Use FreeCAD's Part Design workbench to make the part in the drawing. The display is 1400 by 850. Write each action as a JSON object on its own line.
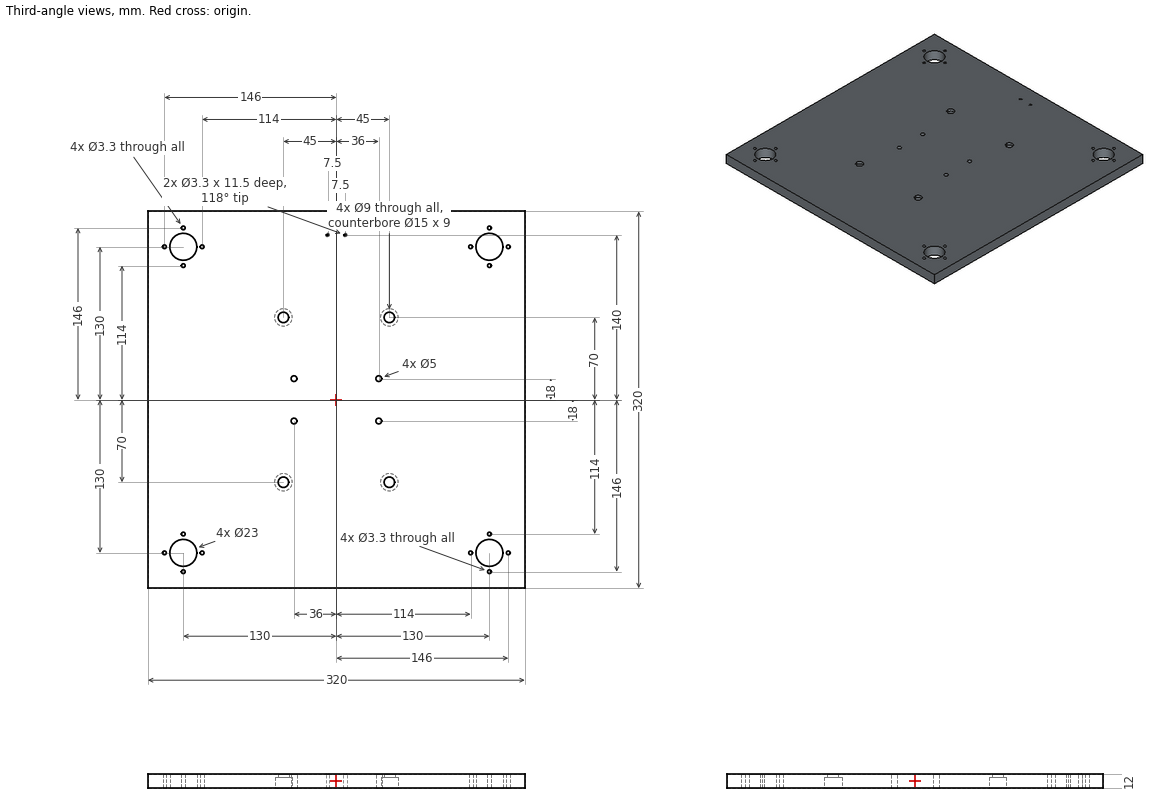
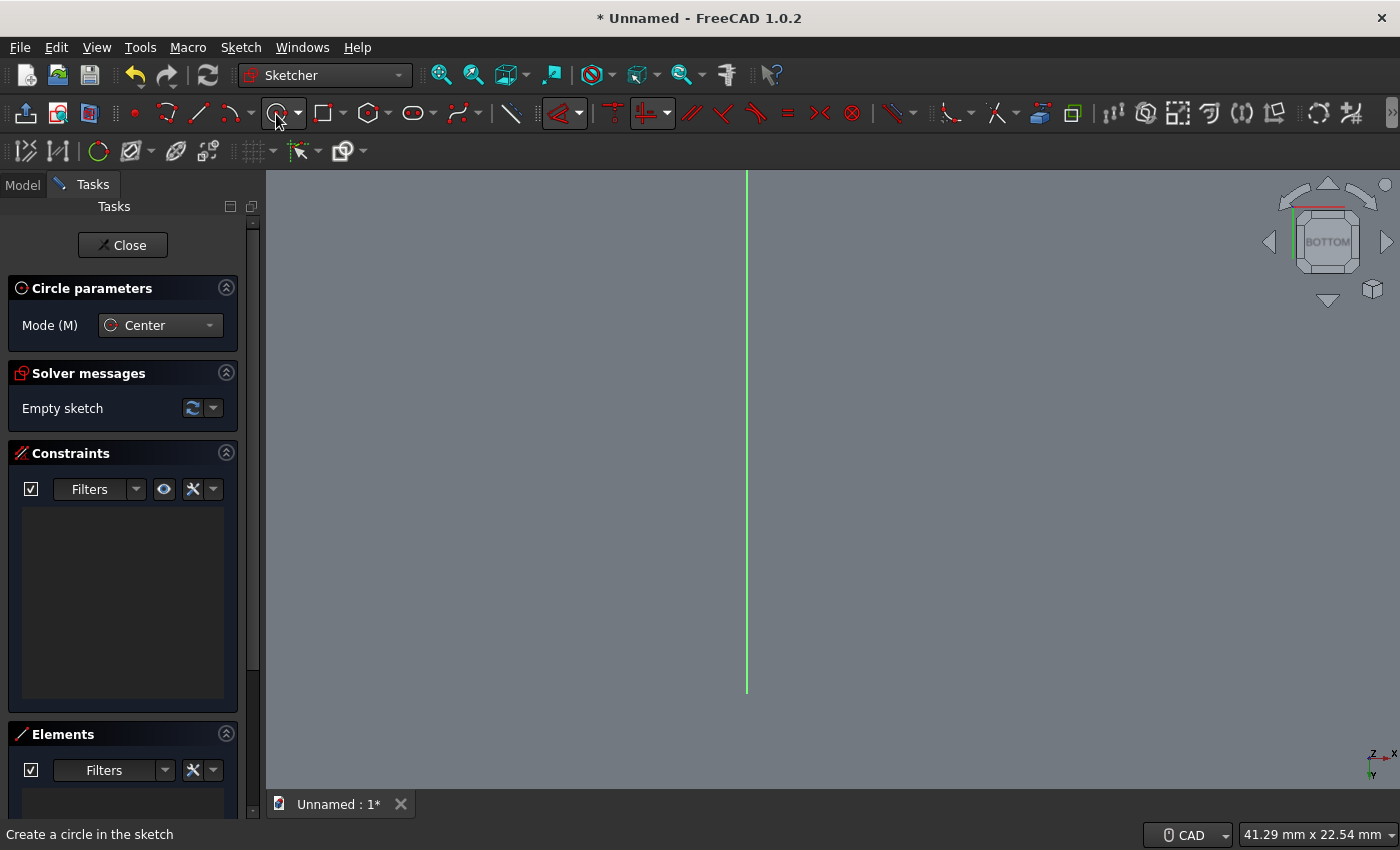
{"action": "left_click", "coordinate": [953, 463]}
{"action": "mouse_move", "coordinate": [985, 431]}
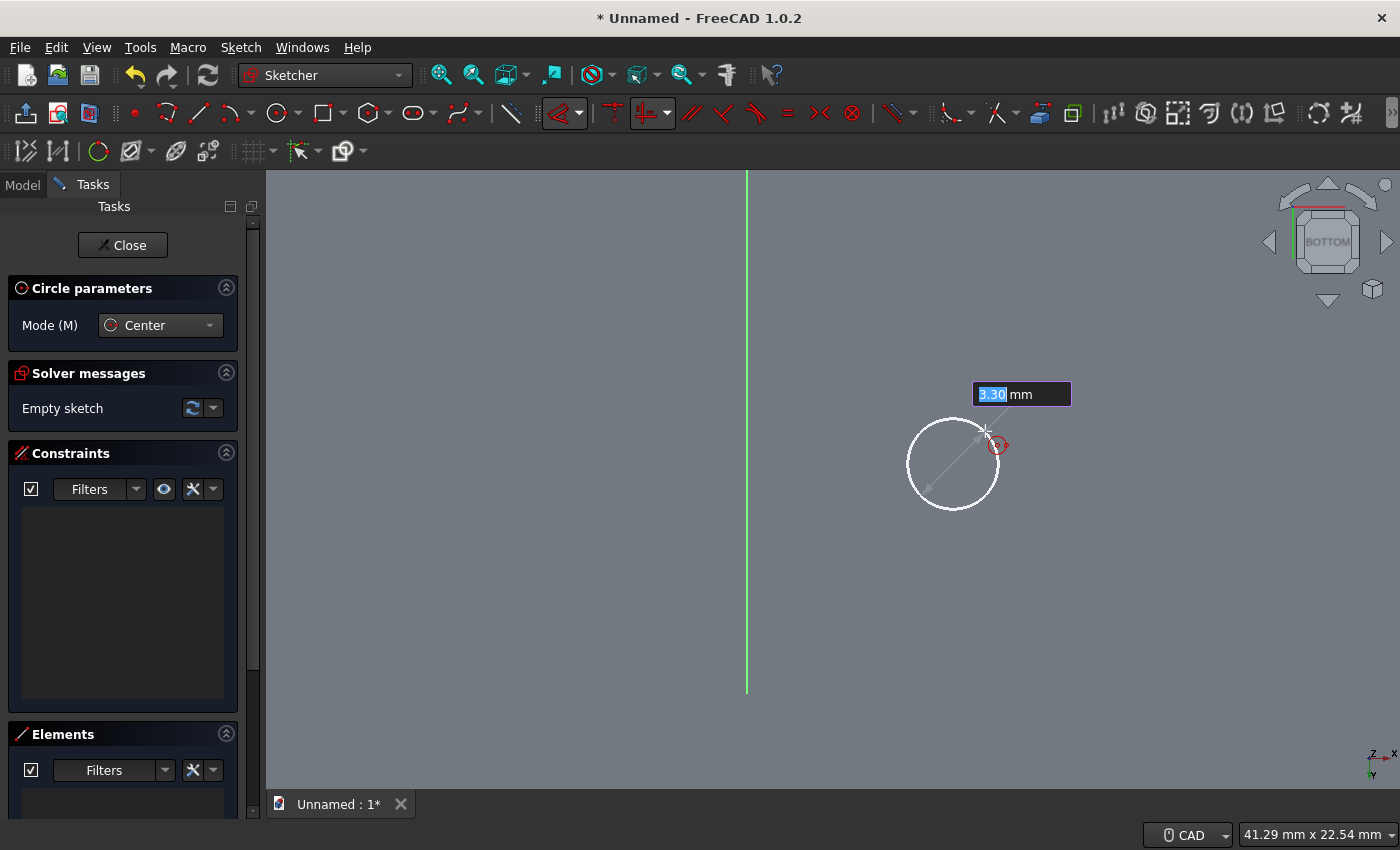
{"action": "type", "text": "3.3"}
{"action": "key", "text": "Return"}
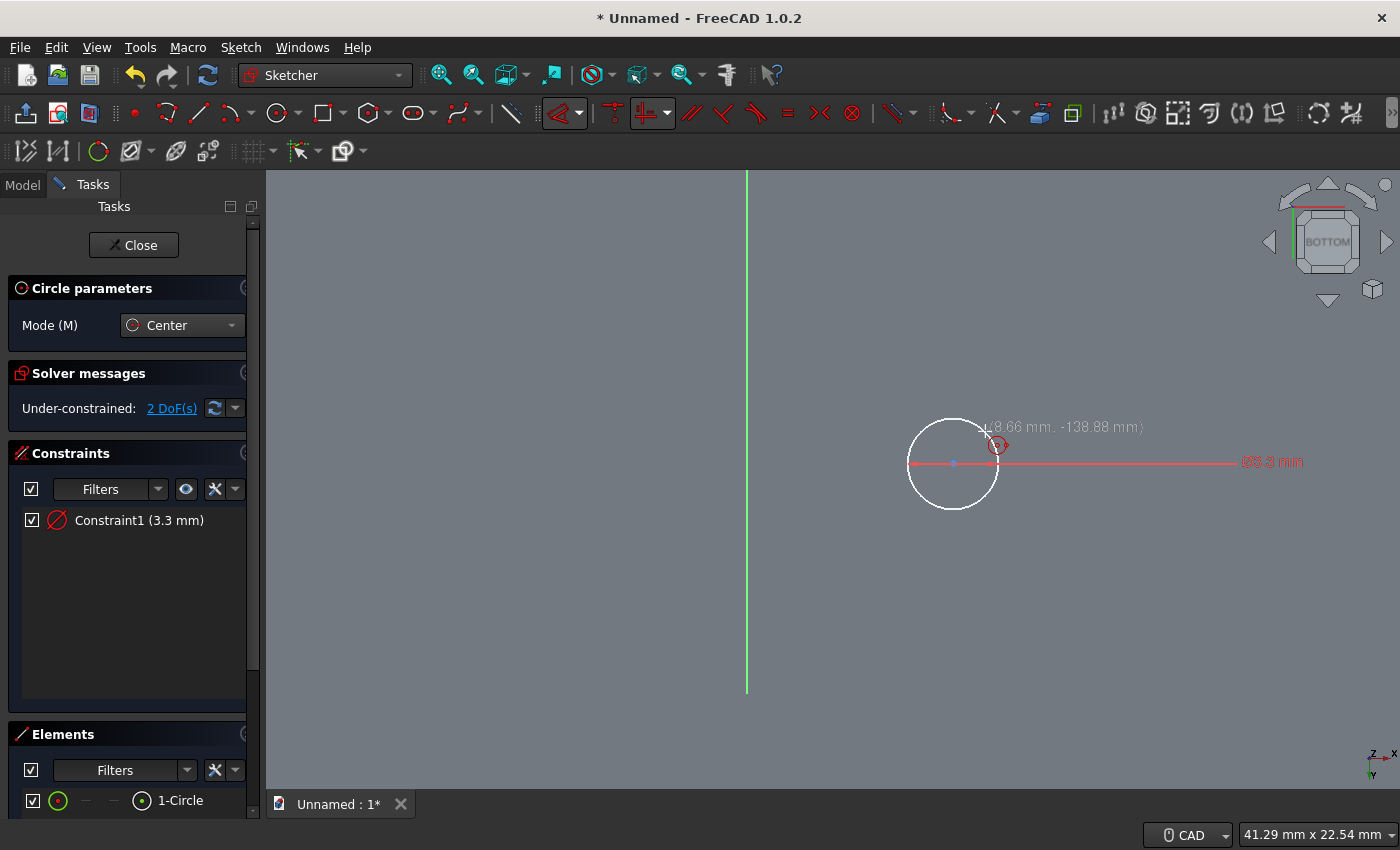
{"action": "left_click", "coordinate": [541, 463]}
{"action": "mouse_move", "coordinate": [573, 431]}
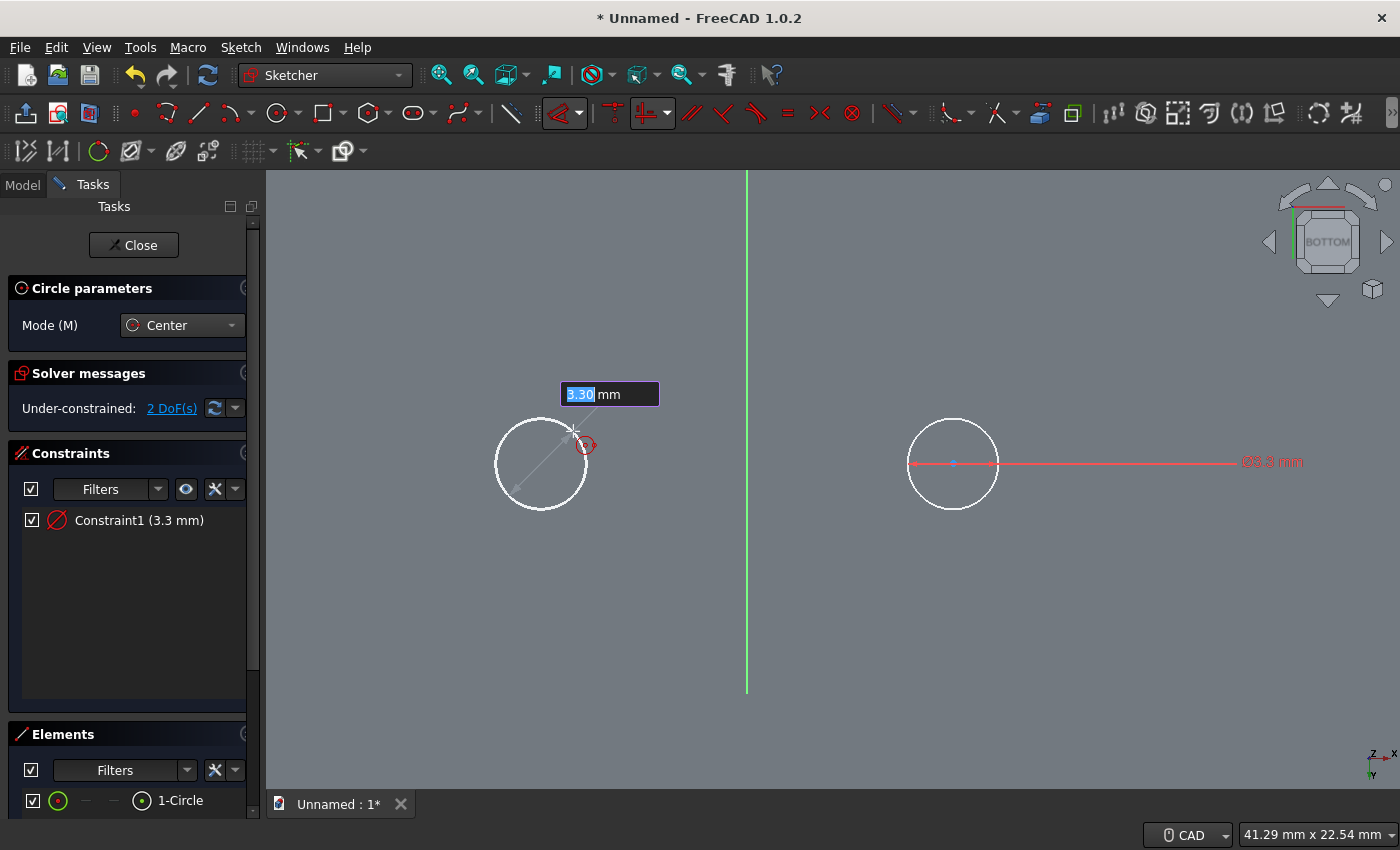
{"action": "type", "text": "3.3"}
{"action": "key", "text": "Return"}
{"action": "key", "text": "Escape"}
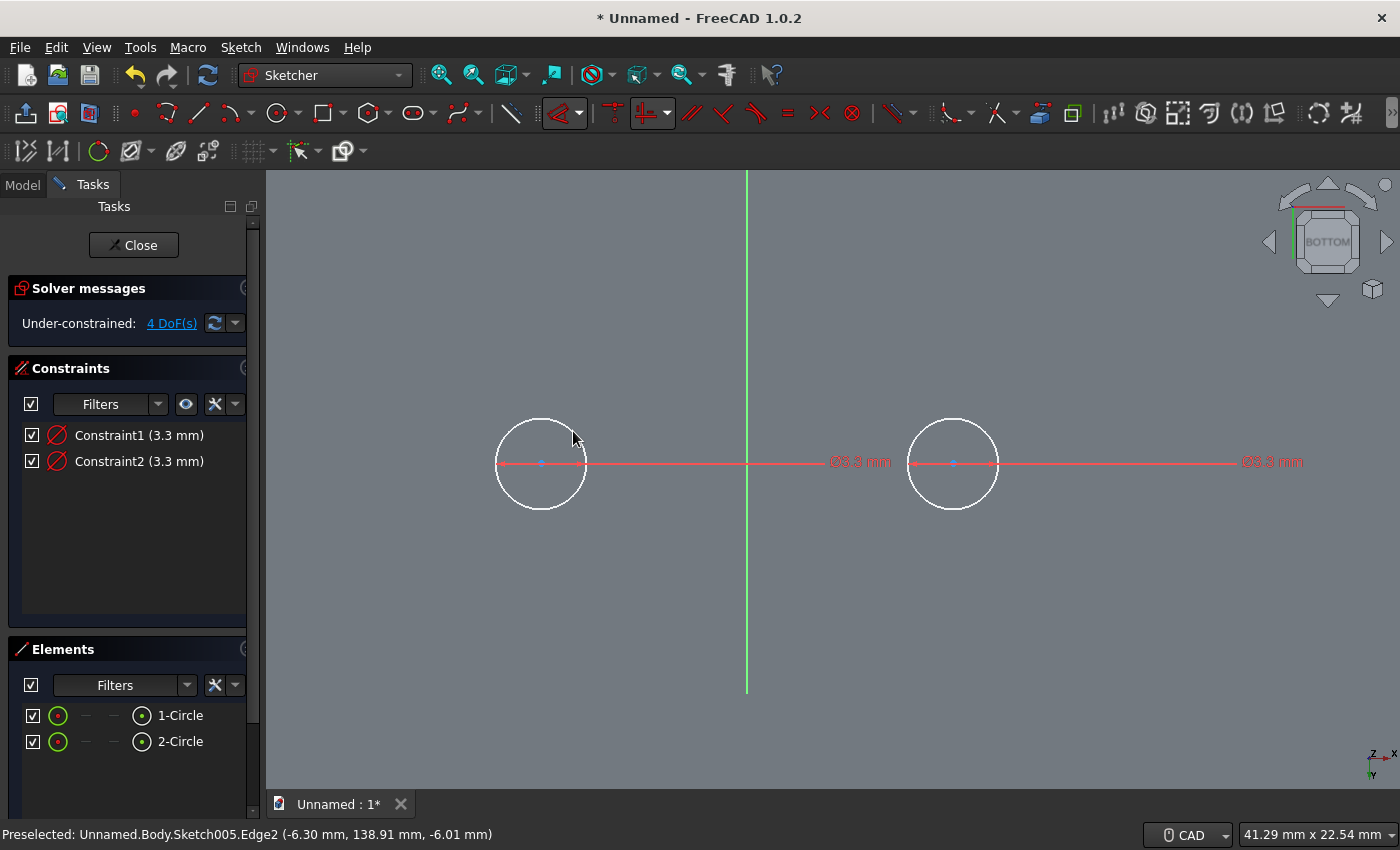
{"action": "left_click", "coordinate": [953, 464]}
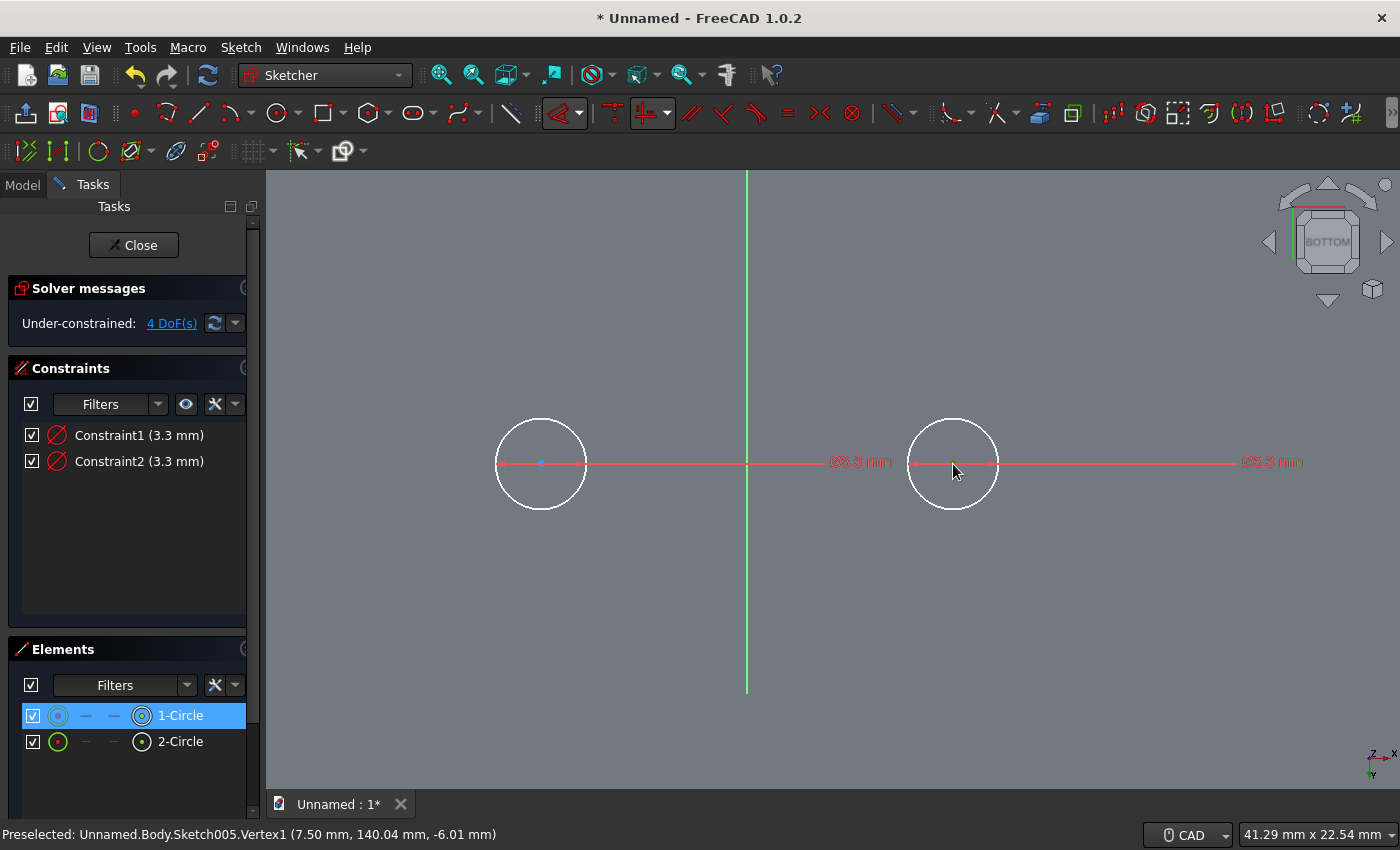
{"action": "left_click", "coordinate": [541, 464]}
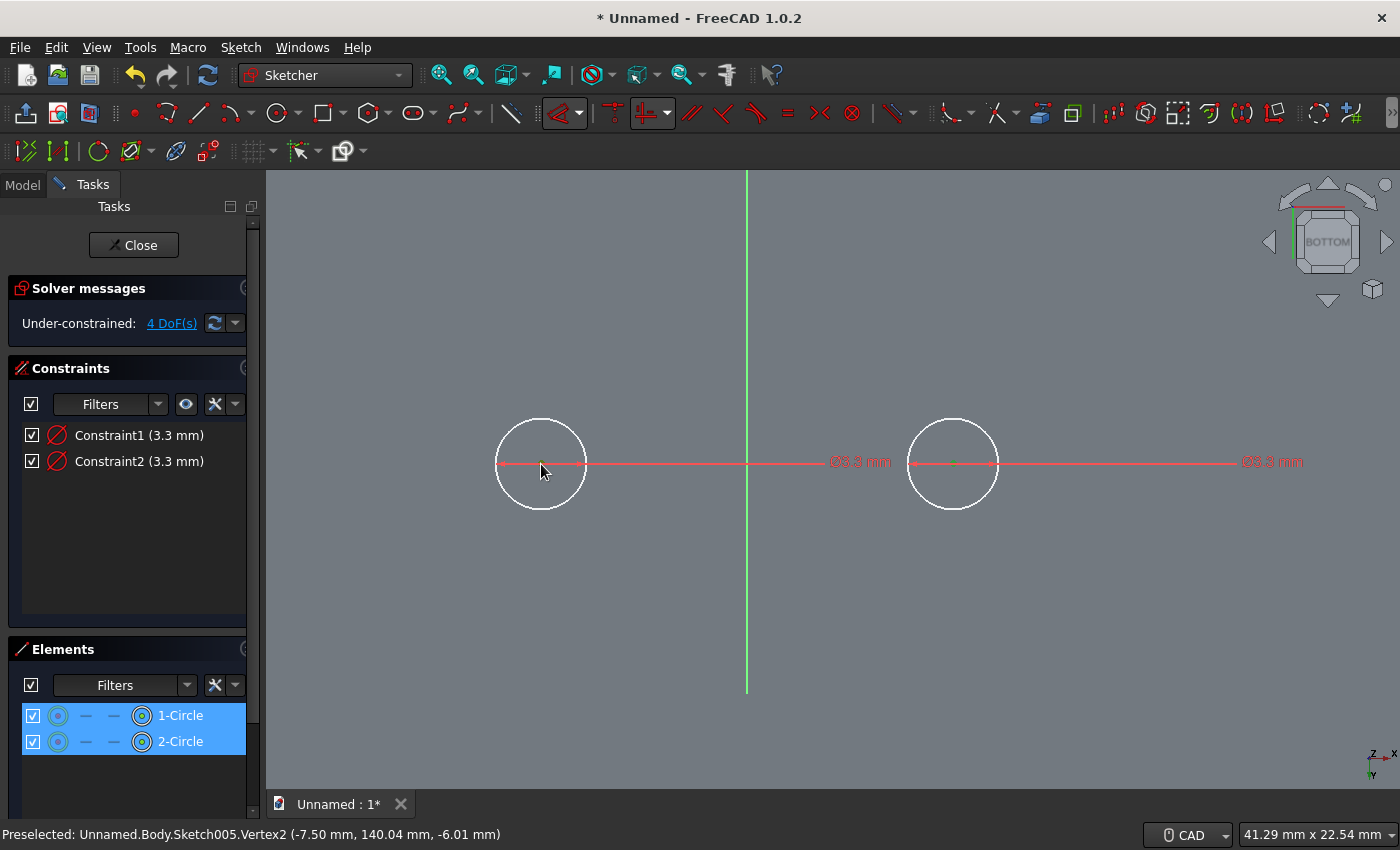
{"action": "left_click", "coordinate": [670, 114]}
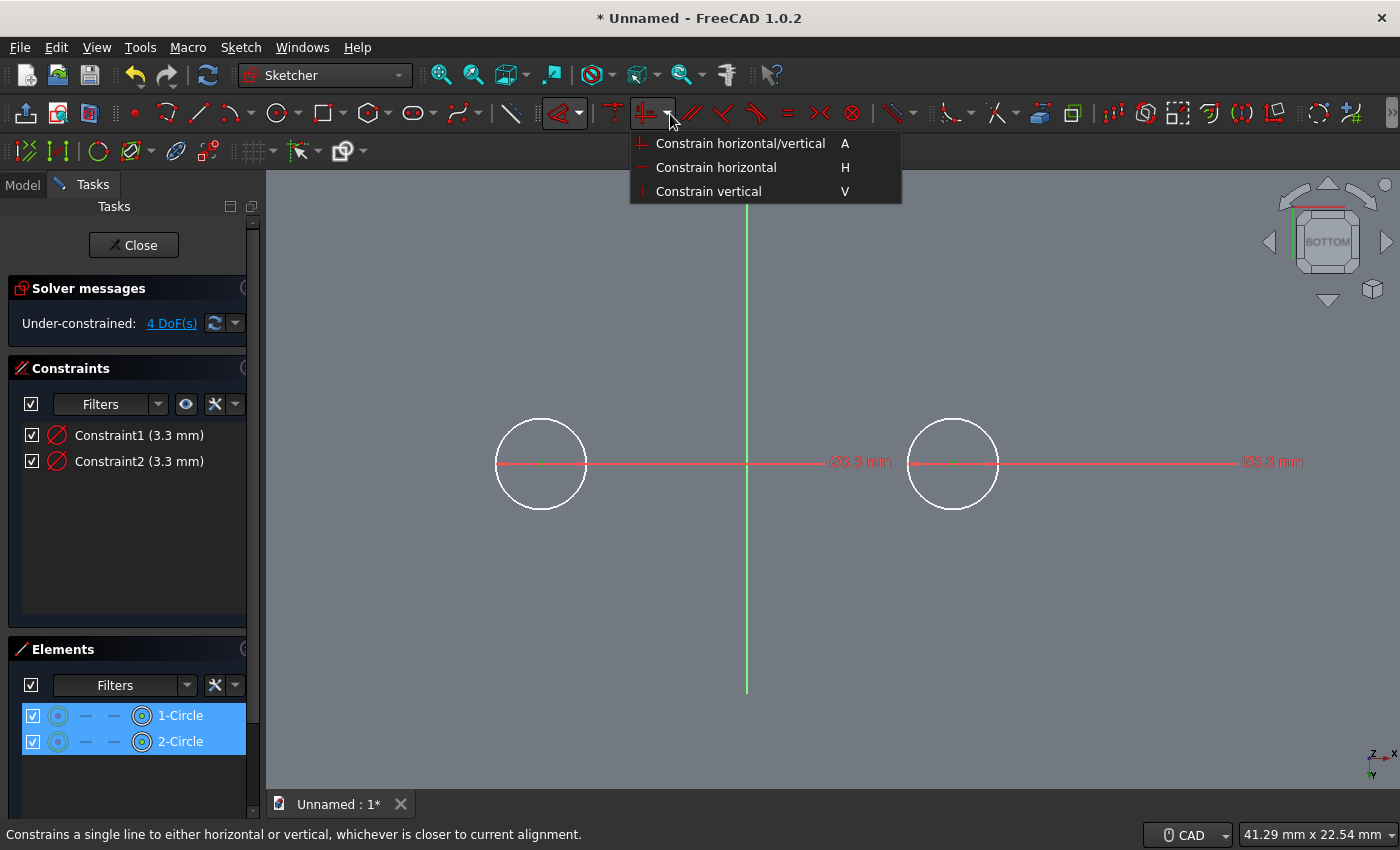
{"action": "left_click", "coordinate": [766, 167]}